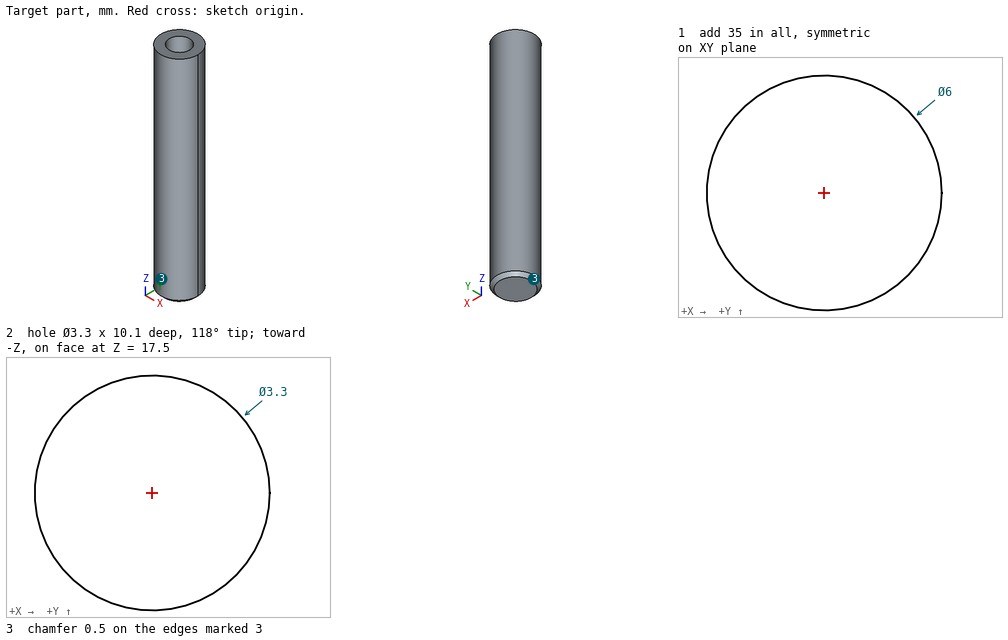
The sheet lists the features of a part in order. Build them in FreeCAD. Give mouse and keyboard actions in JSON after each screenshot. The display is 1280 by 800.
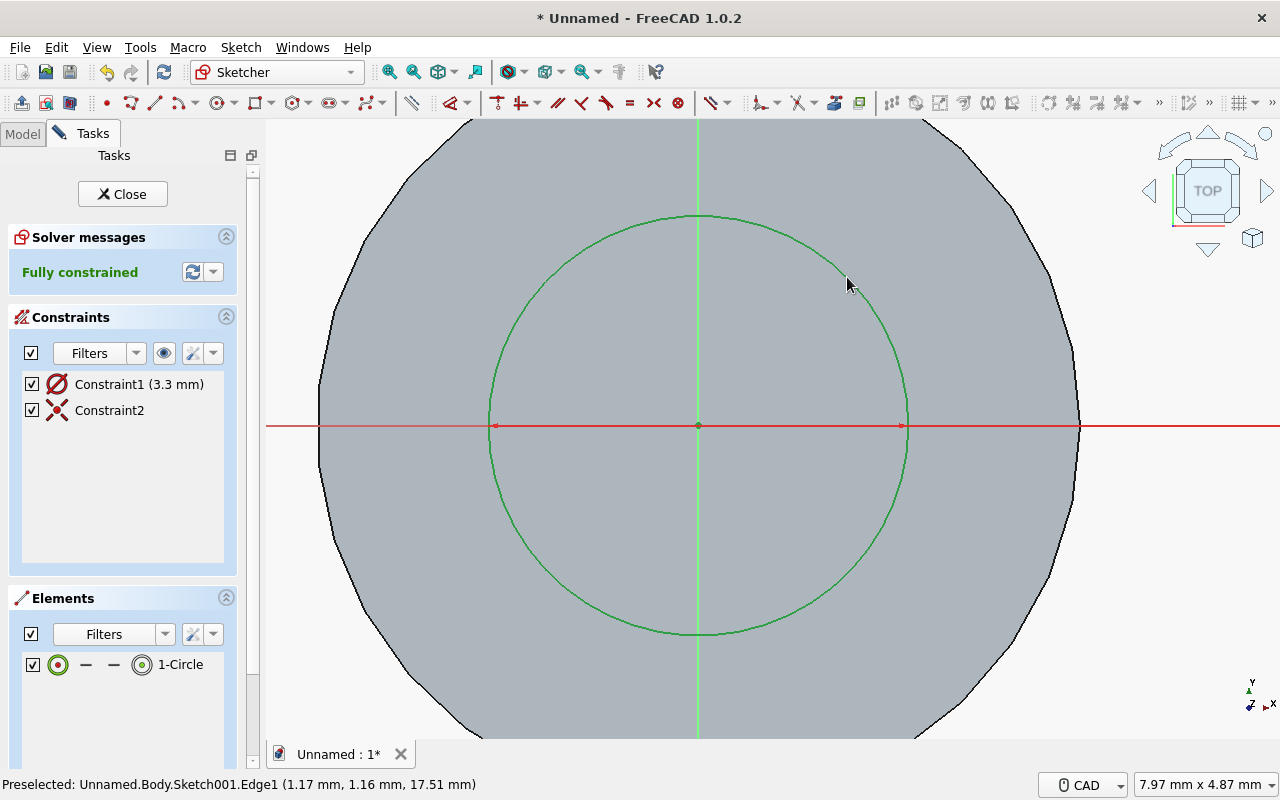
{"action": "left_click", "coordinate": [123, 194]}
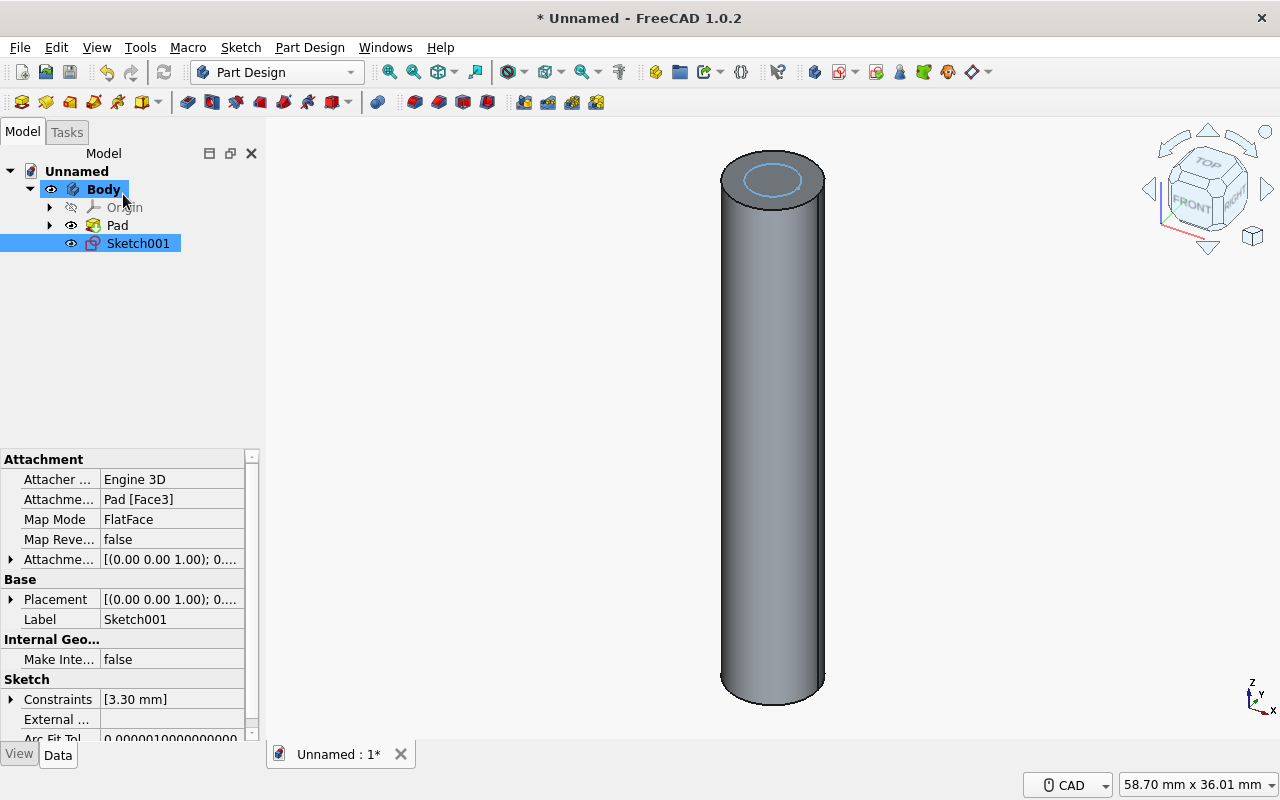
{"action": "left_click", "coordinate": [212, 102]}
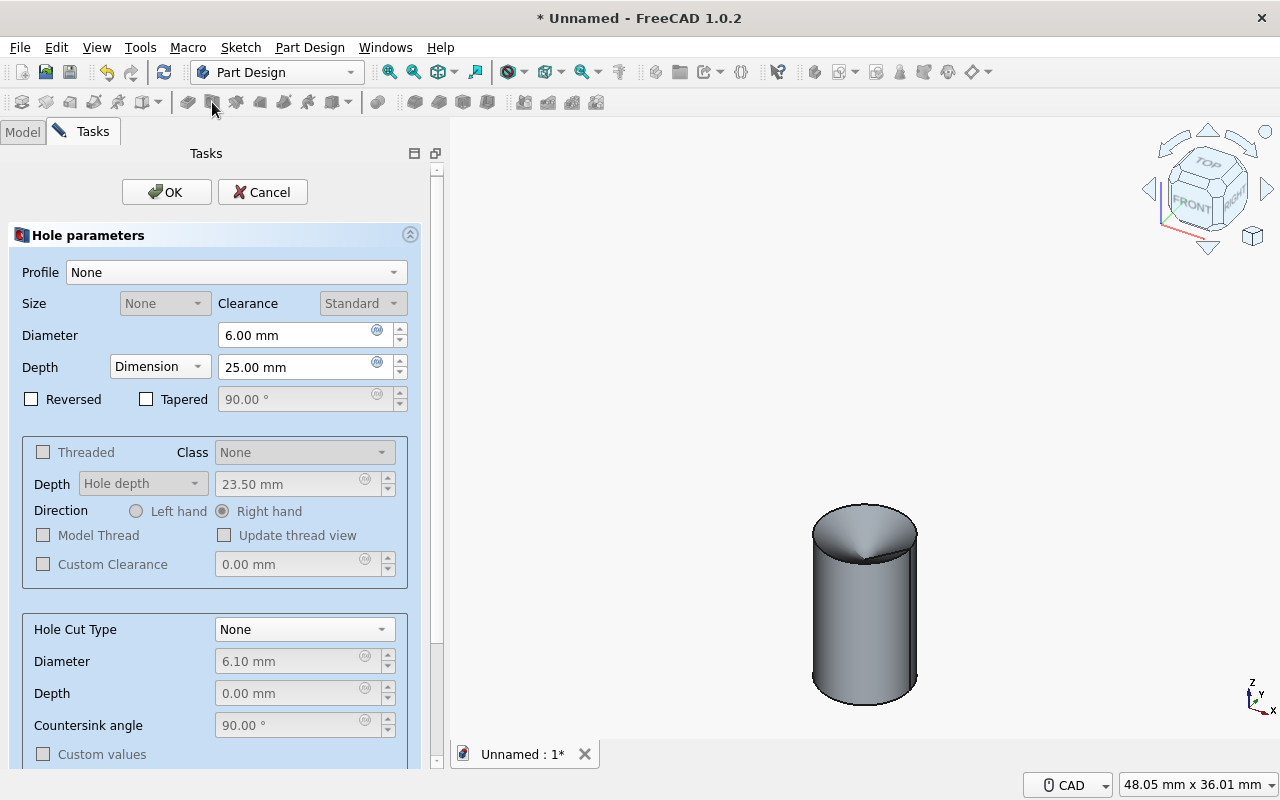
{"action": "triple_click", "coordinate": [305, 335]}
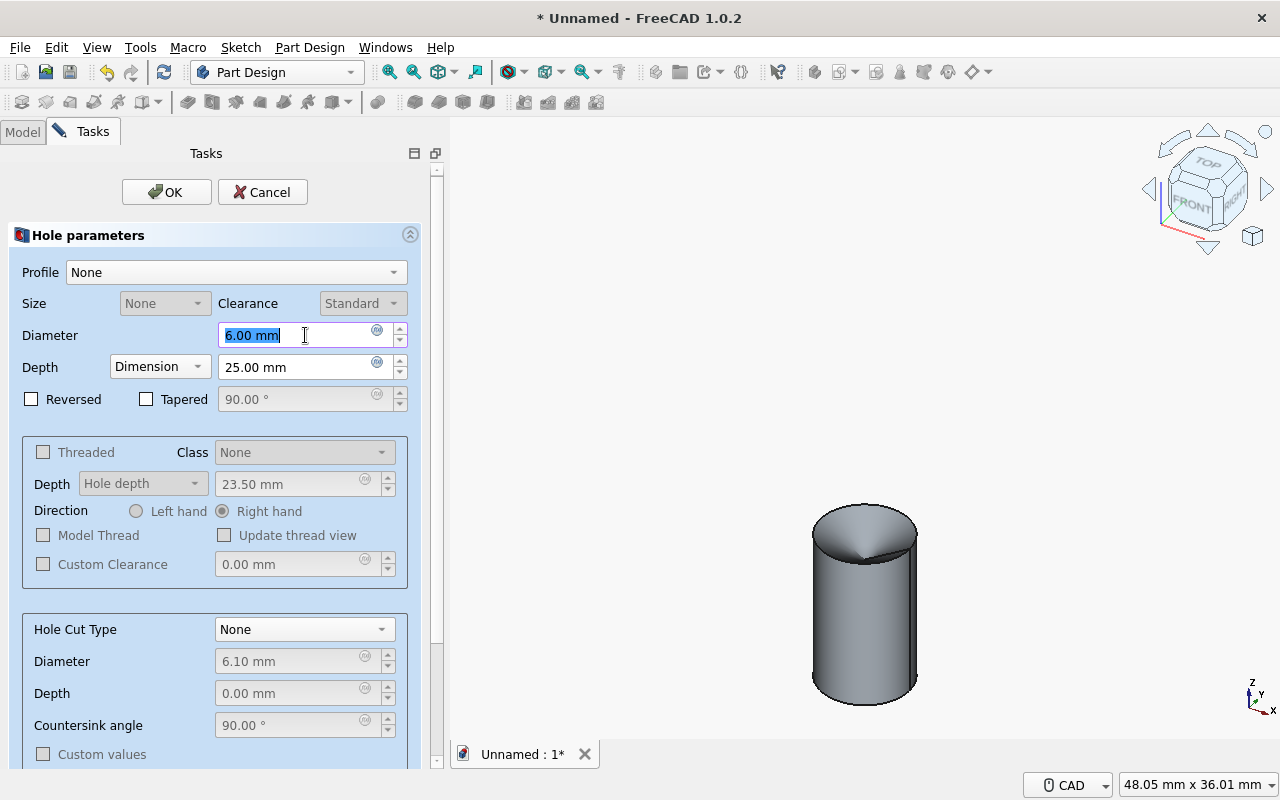
{"action": "type", "text": "3.3"}
{"action": "key", "text": "Tab"}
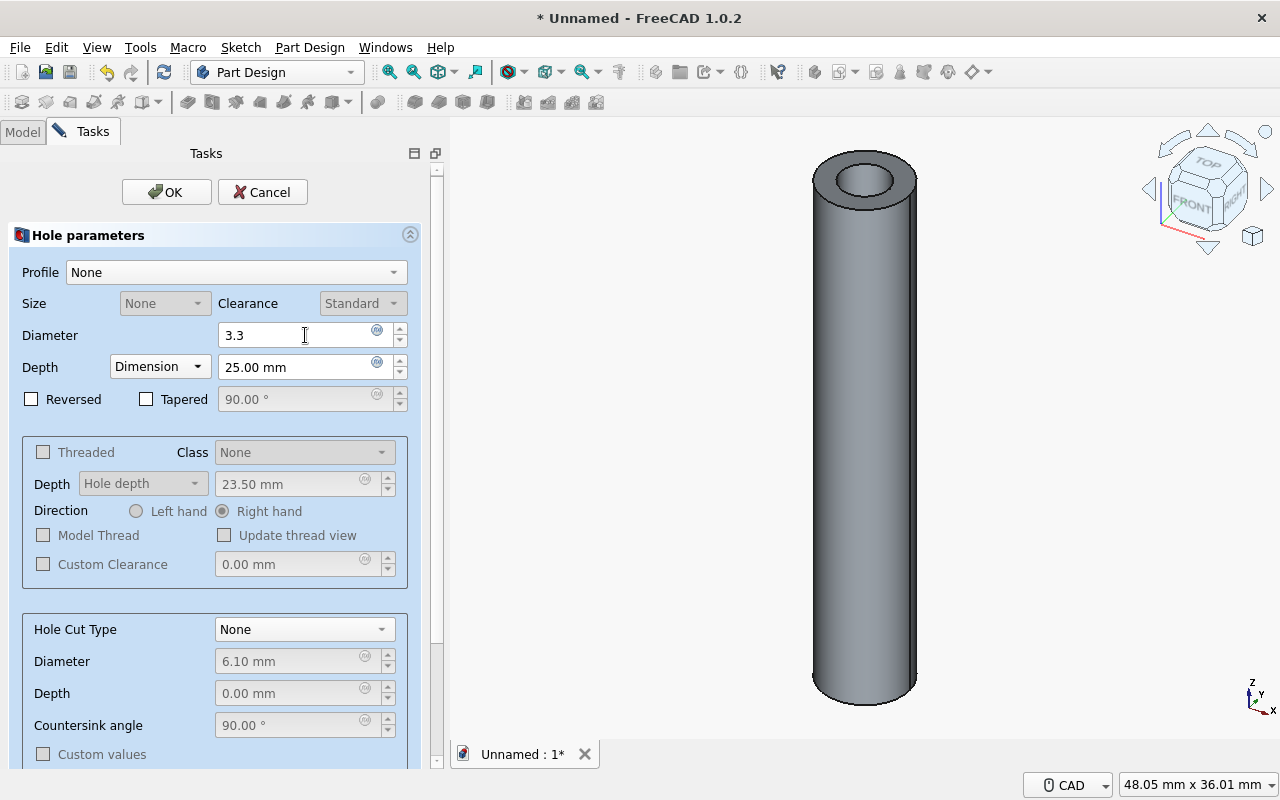
{"action": "triple_click", "coordinate": [305, 367]}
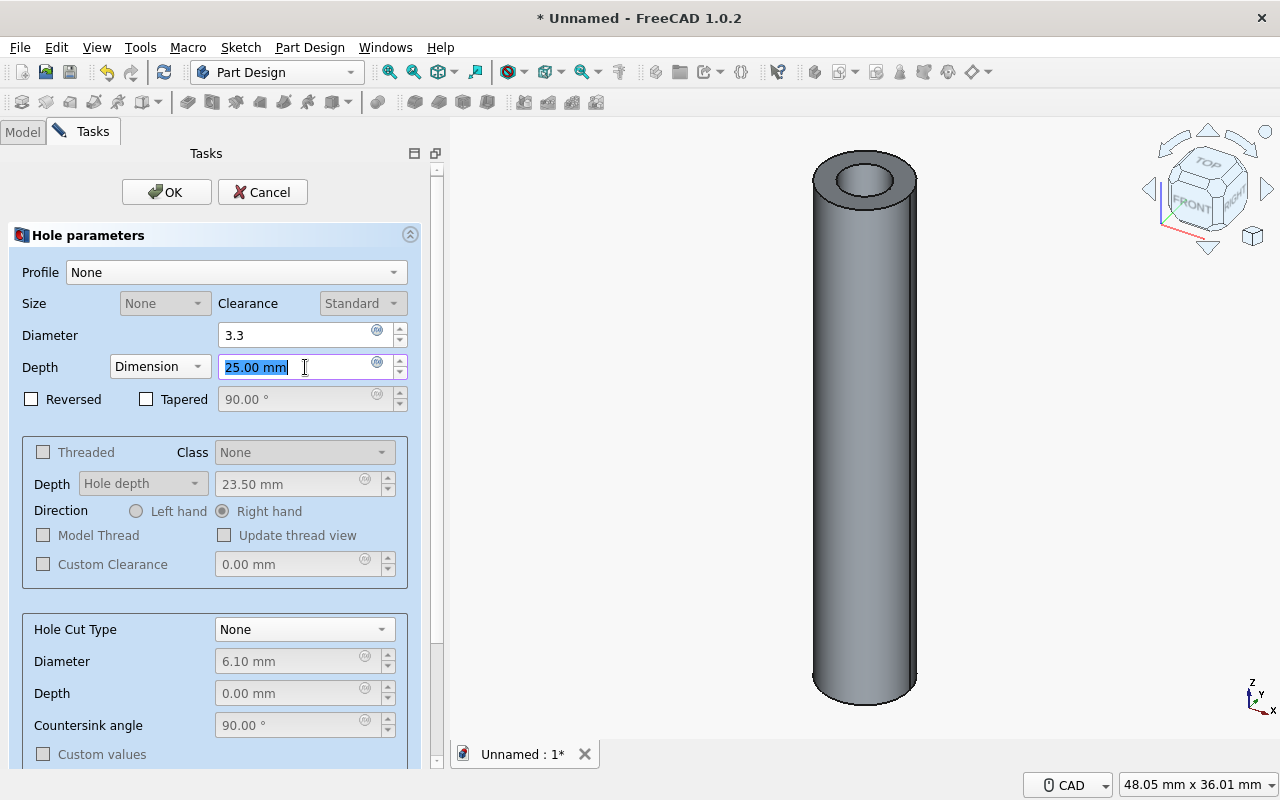
{"action": "type", "text": "10.1"}
{"action": "key", "text": "Tab"}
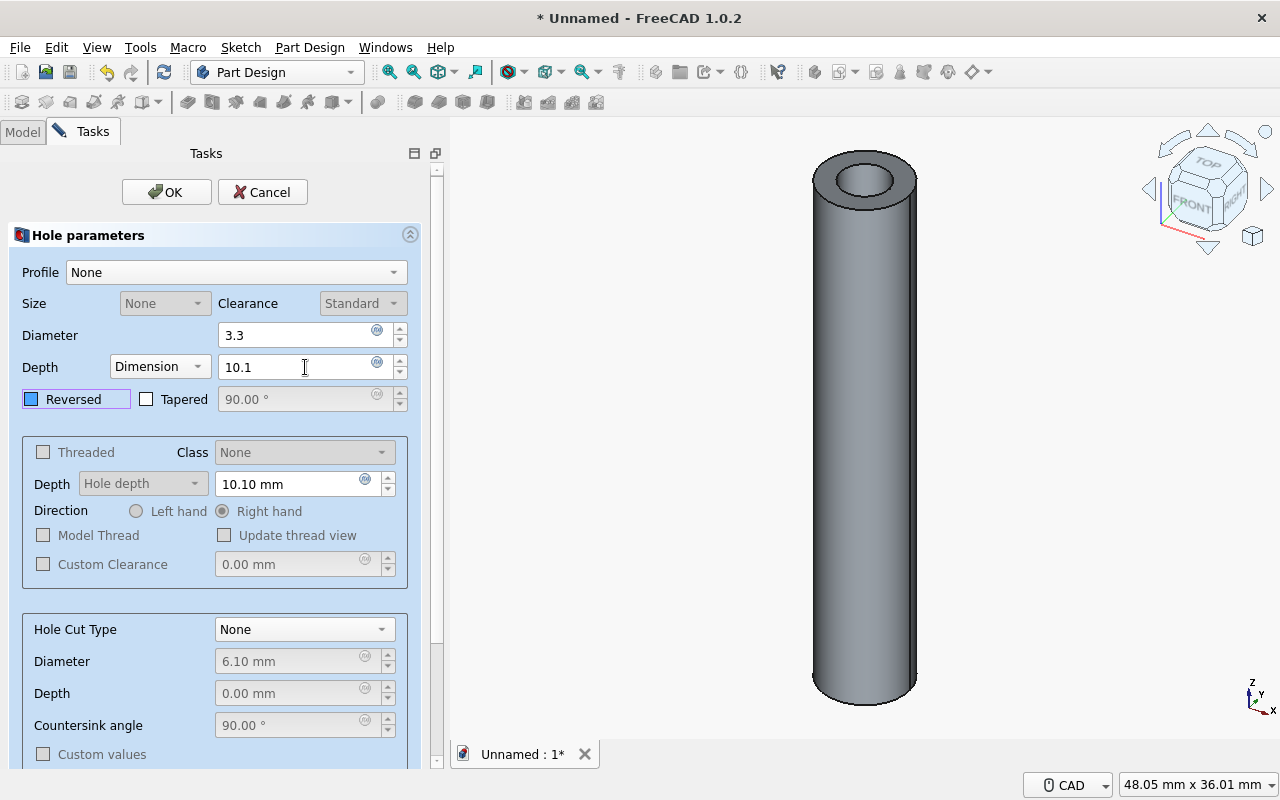
{"action": "left_click", "coordinate": [167, 192]}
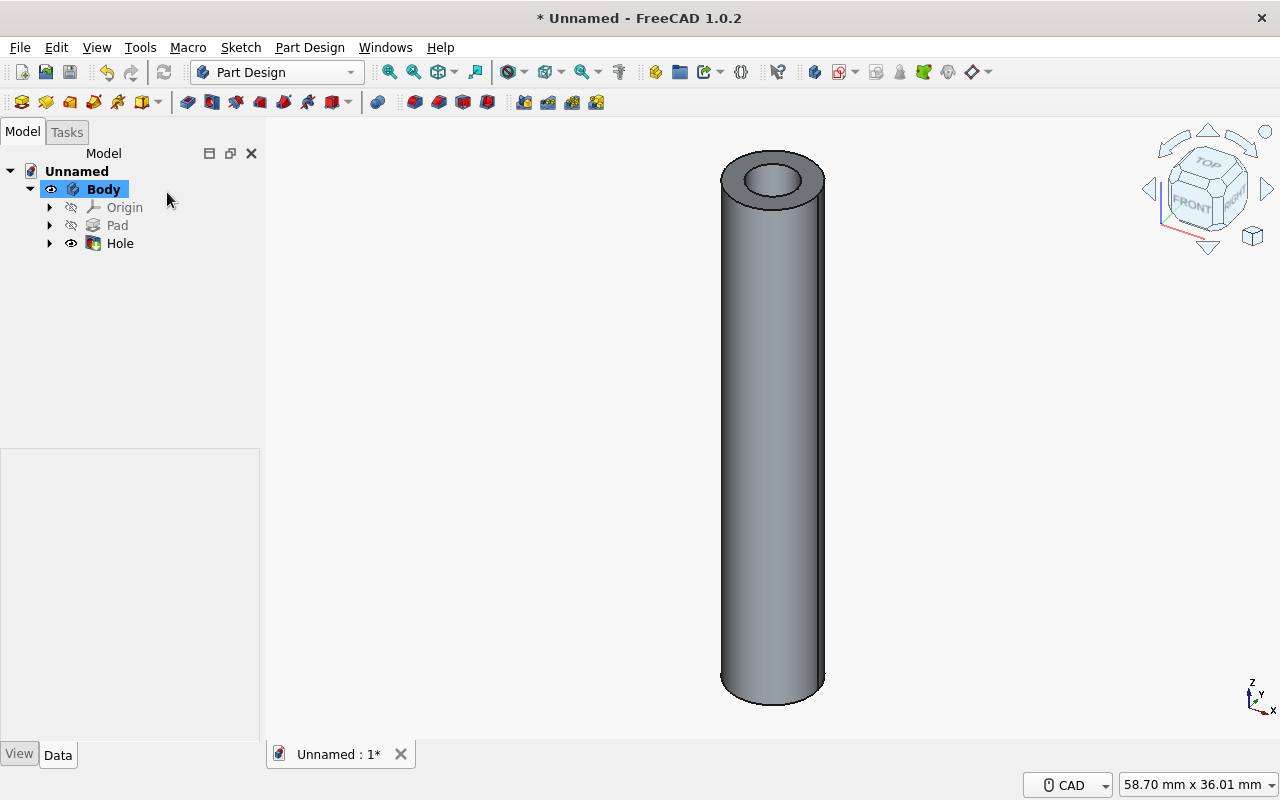
{"action": "key", "text": "0"}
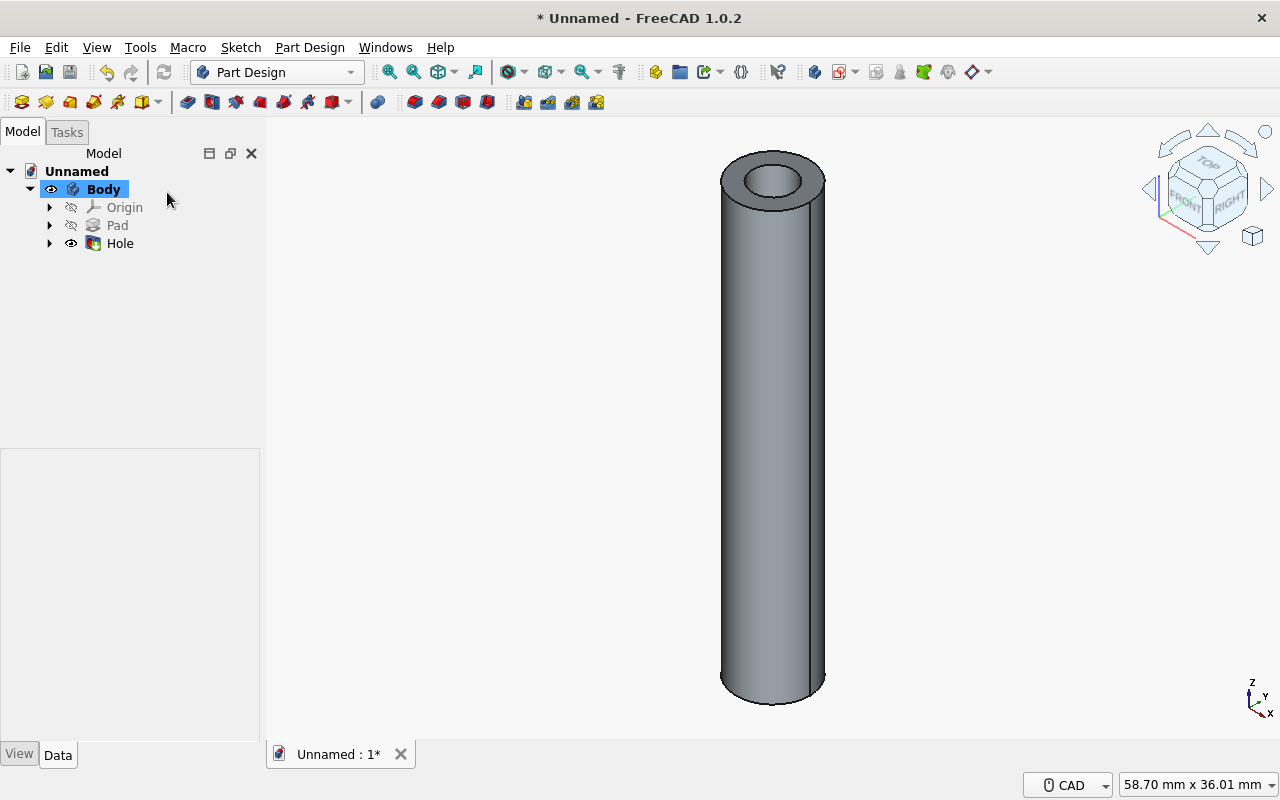
{"action": "key", "text": "2"}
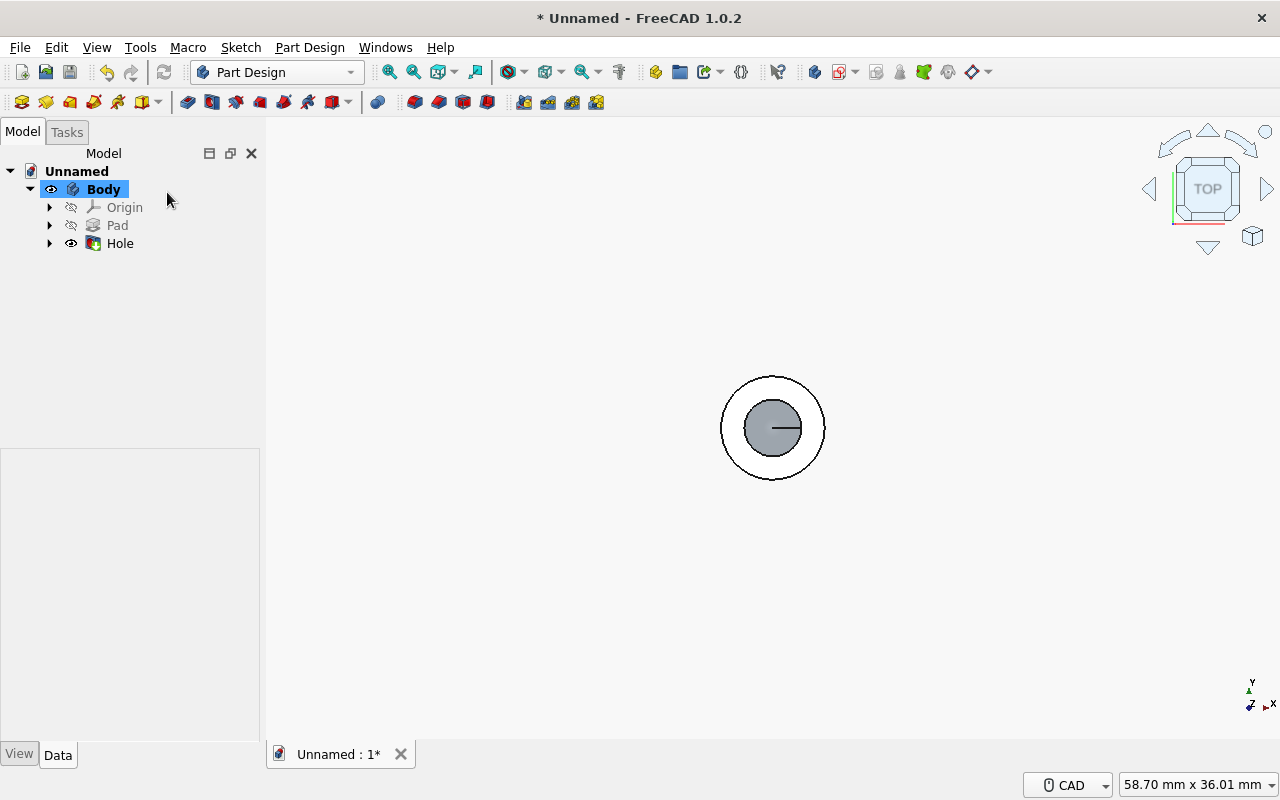
{"action": "left_click", "coordinate": [390, 72]}